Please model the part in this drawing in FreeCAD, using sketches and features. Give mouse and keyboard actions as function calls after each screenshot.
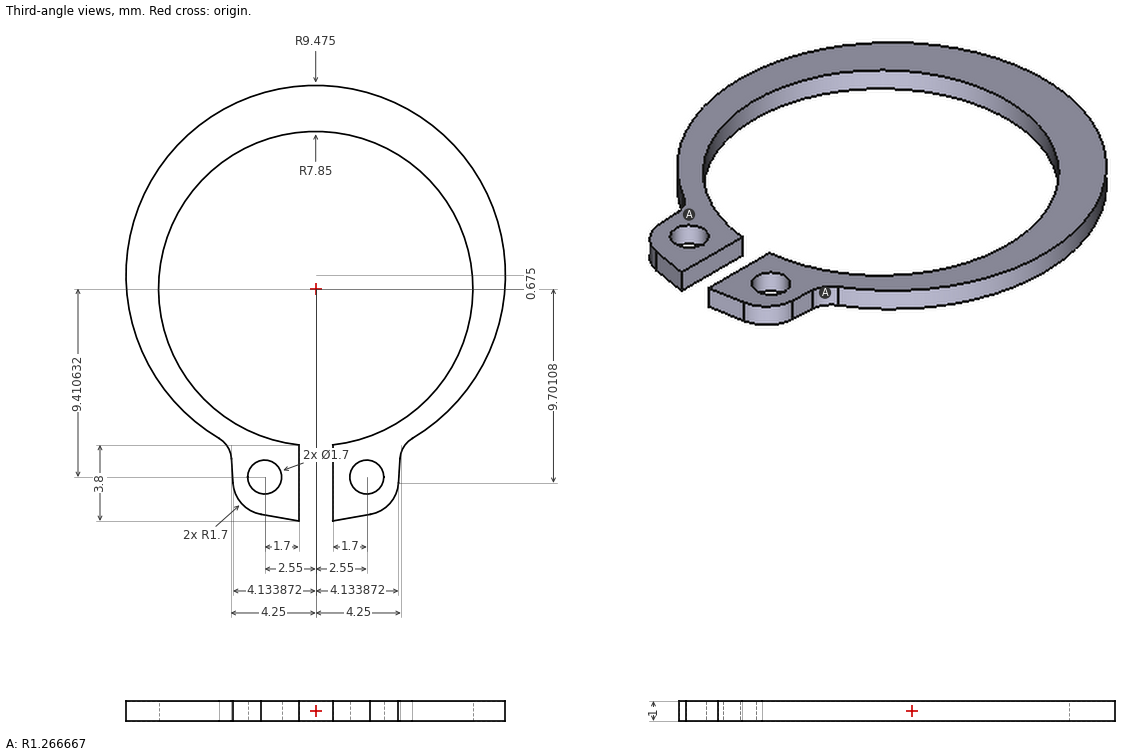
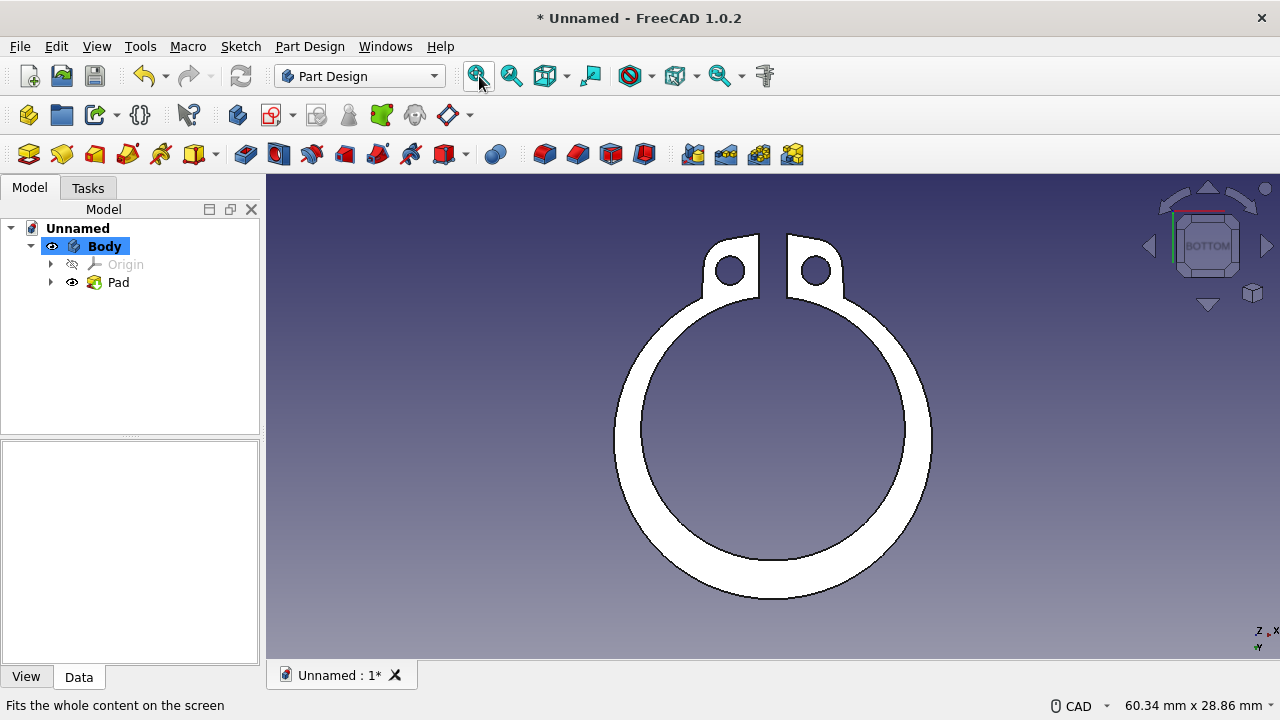
key(4)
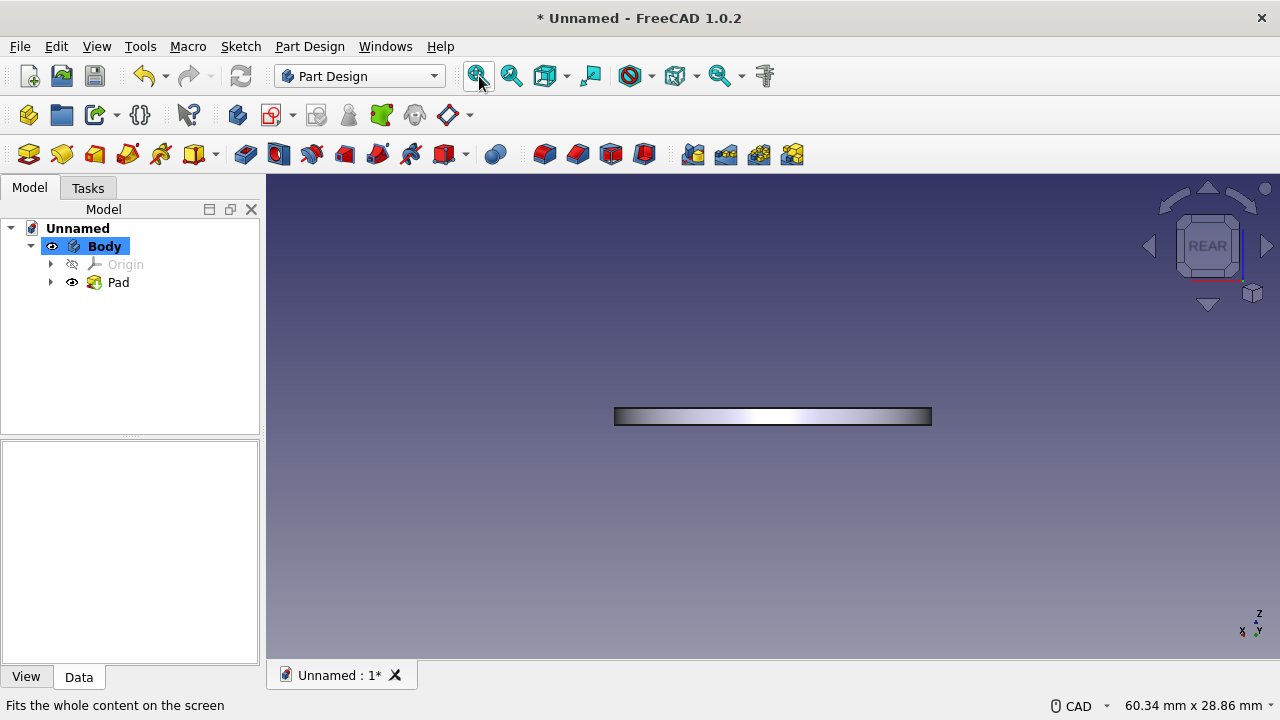
click(479, 76)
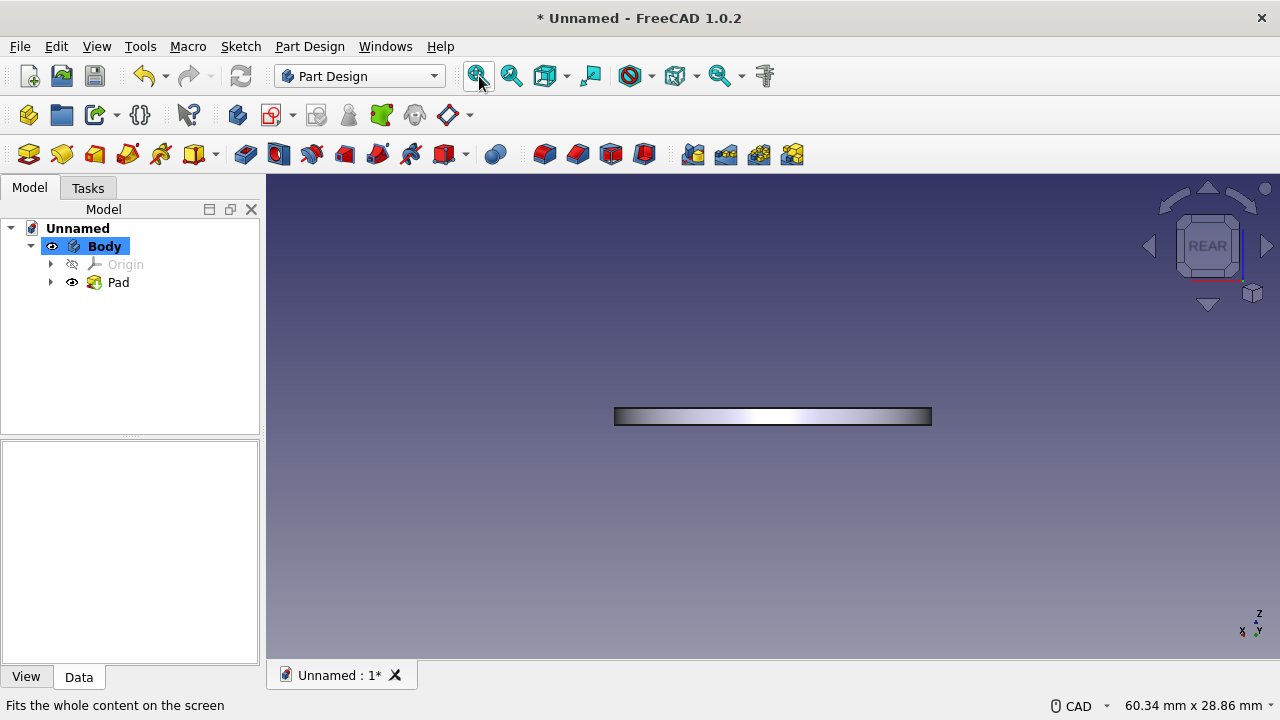
scroll(844, 416, up, 5)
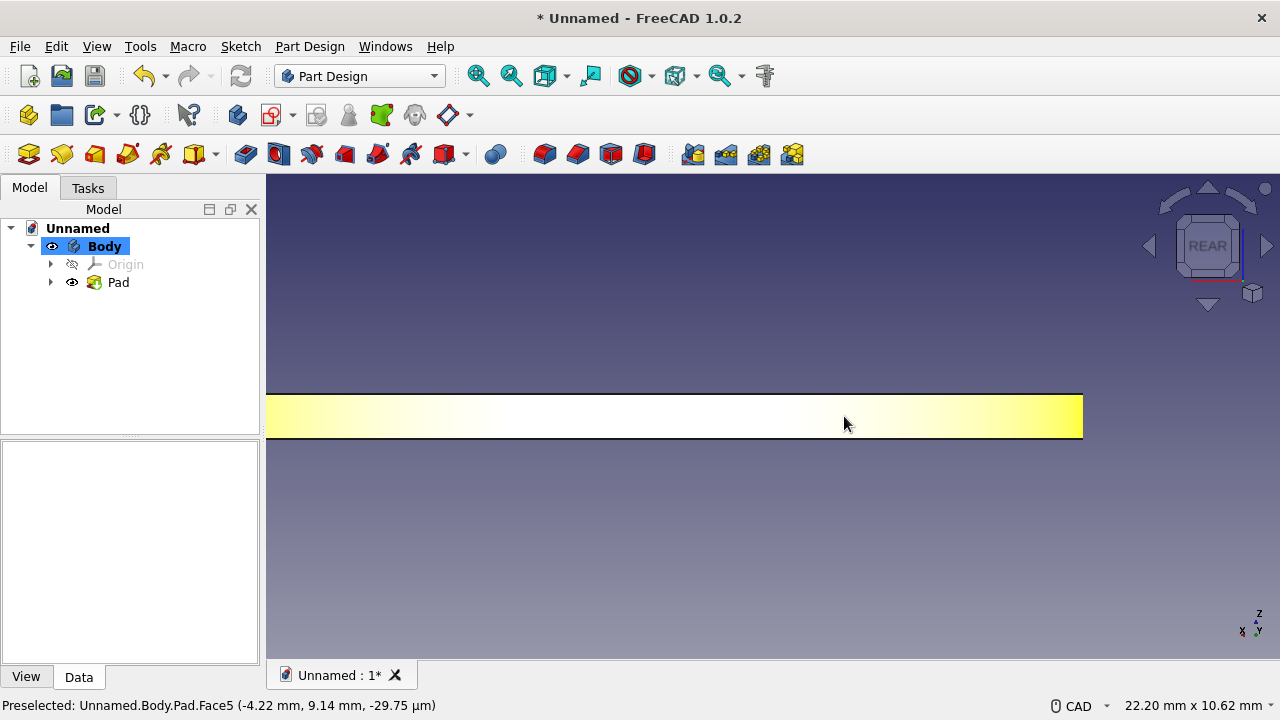
click(479, 76)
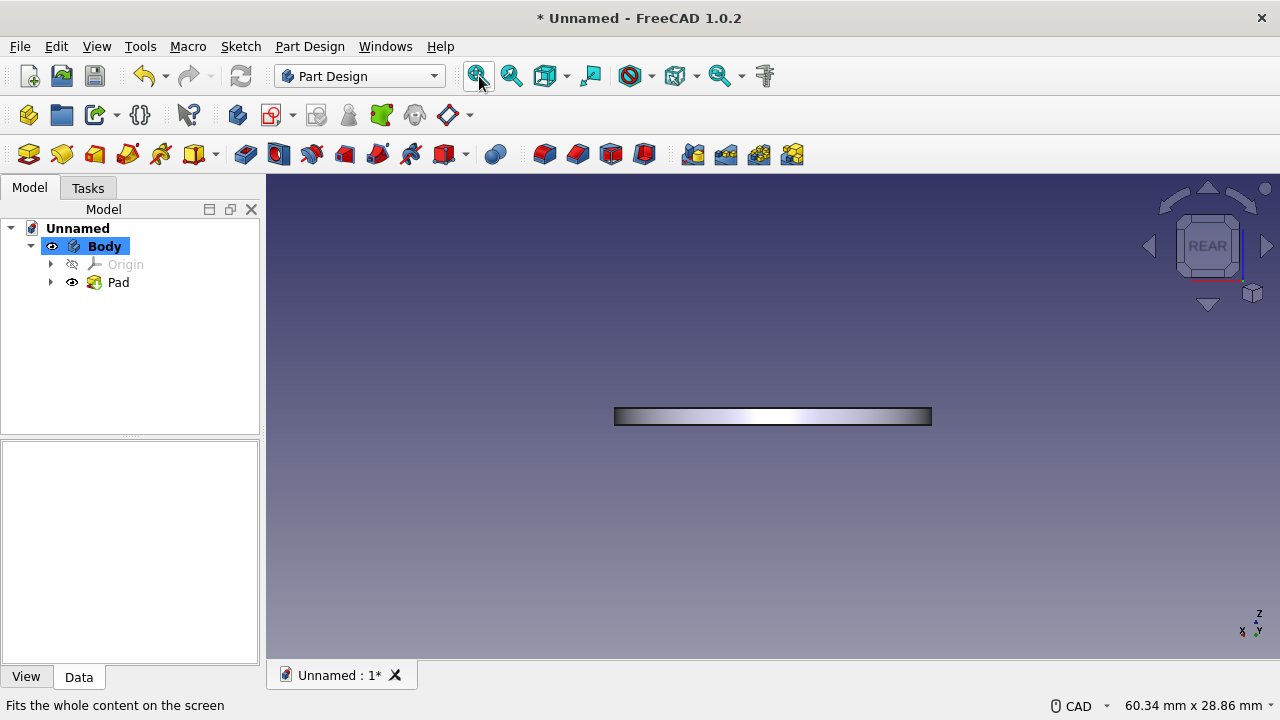
key(6)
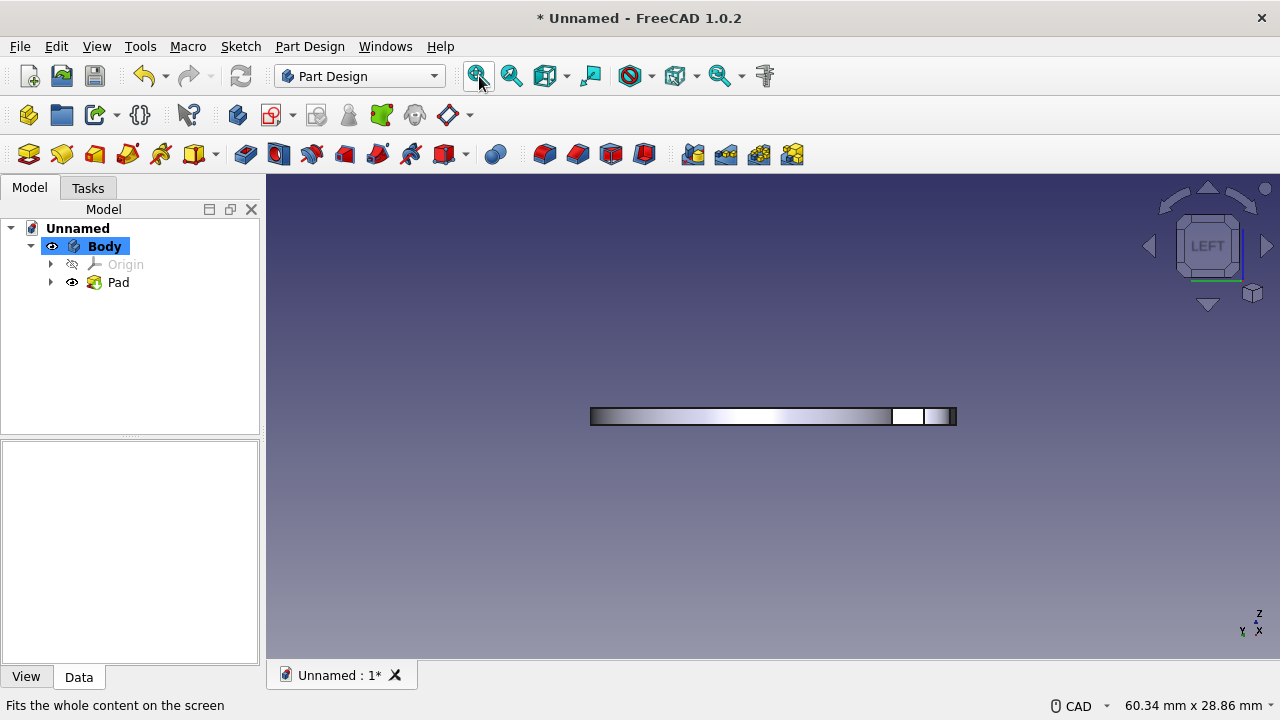
click(479, 76)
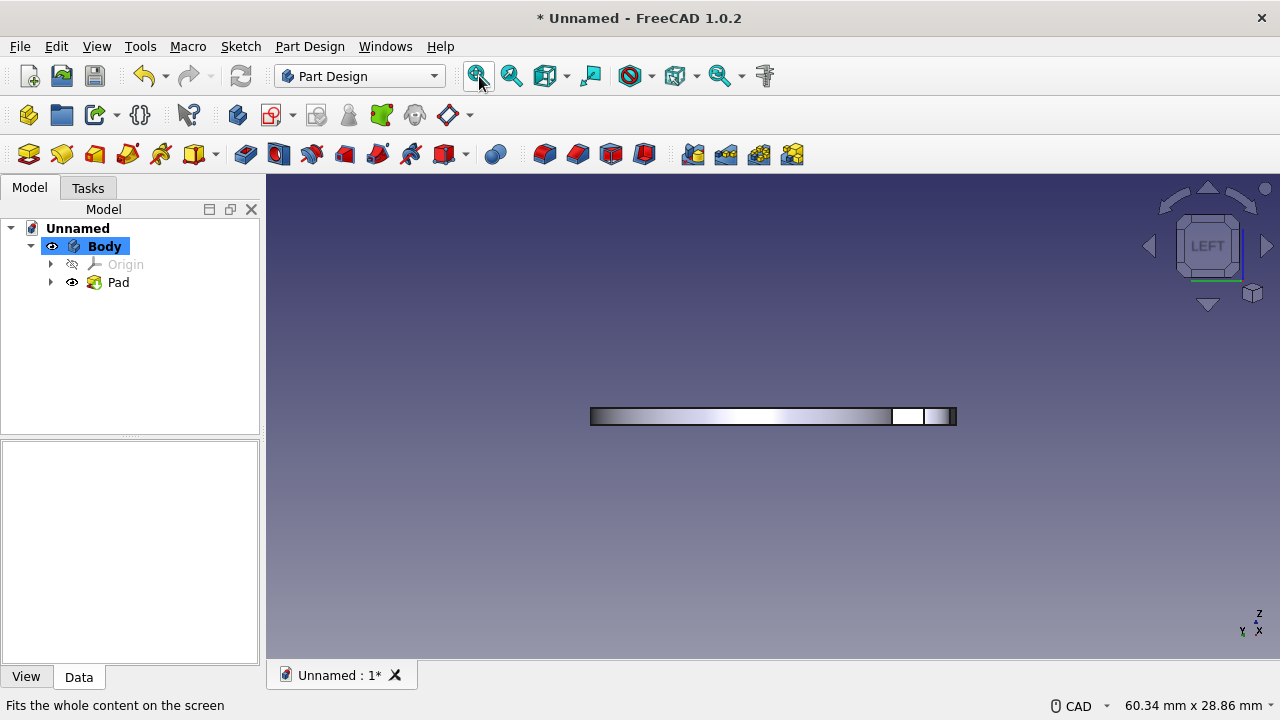
scroll(892, 415, up, 5)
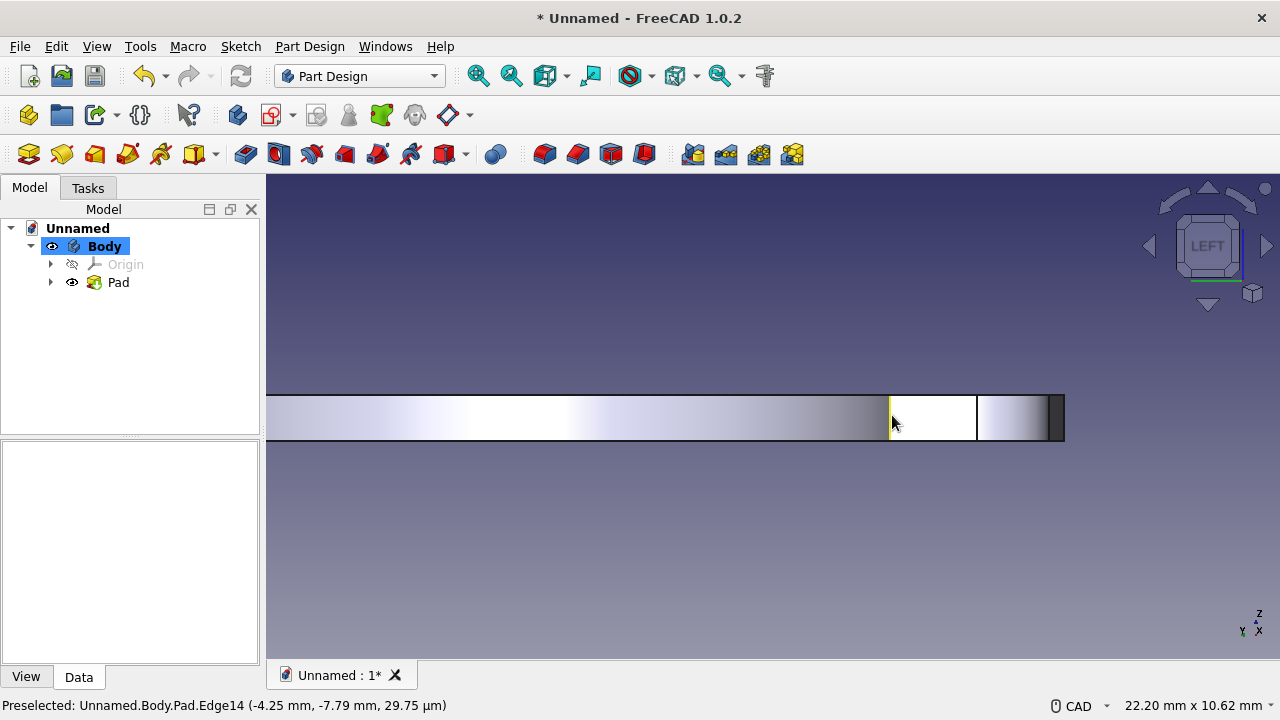
click(479, 76)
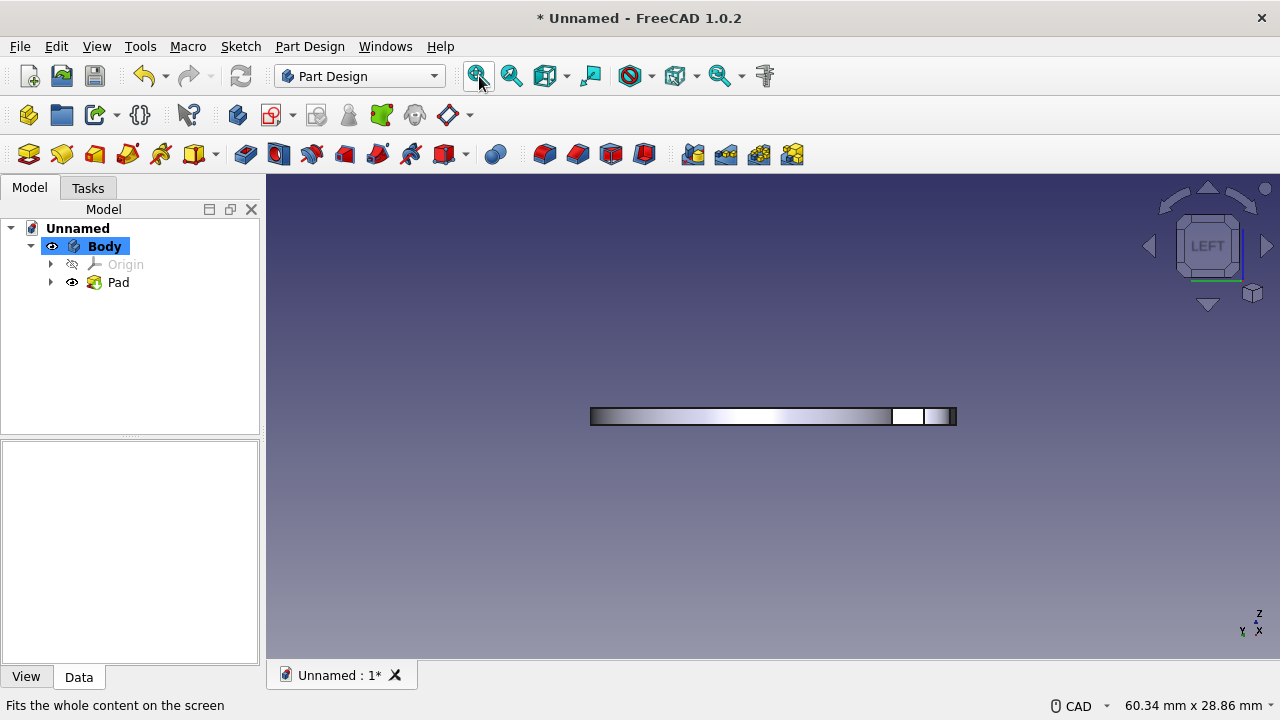
key(v)
key(3)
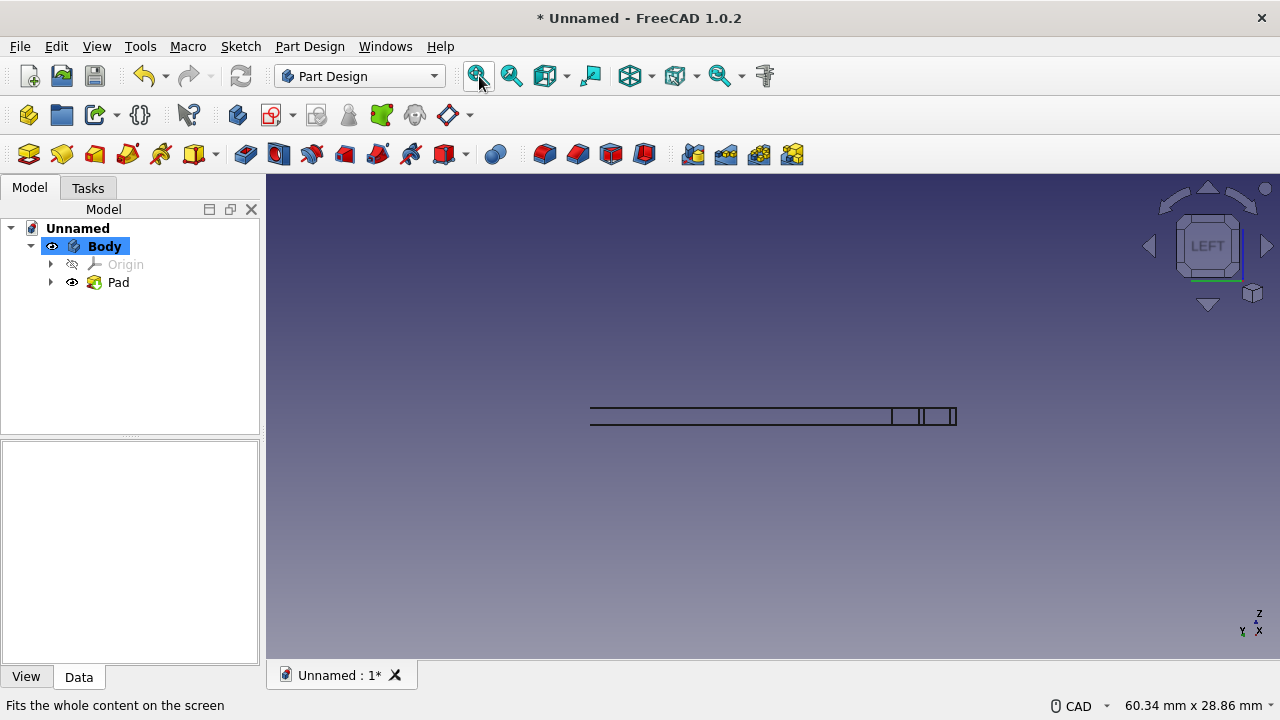
key(0)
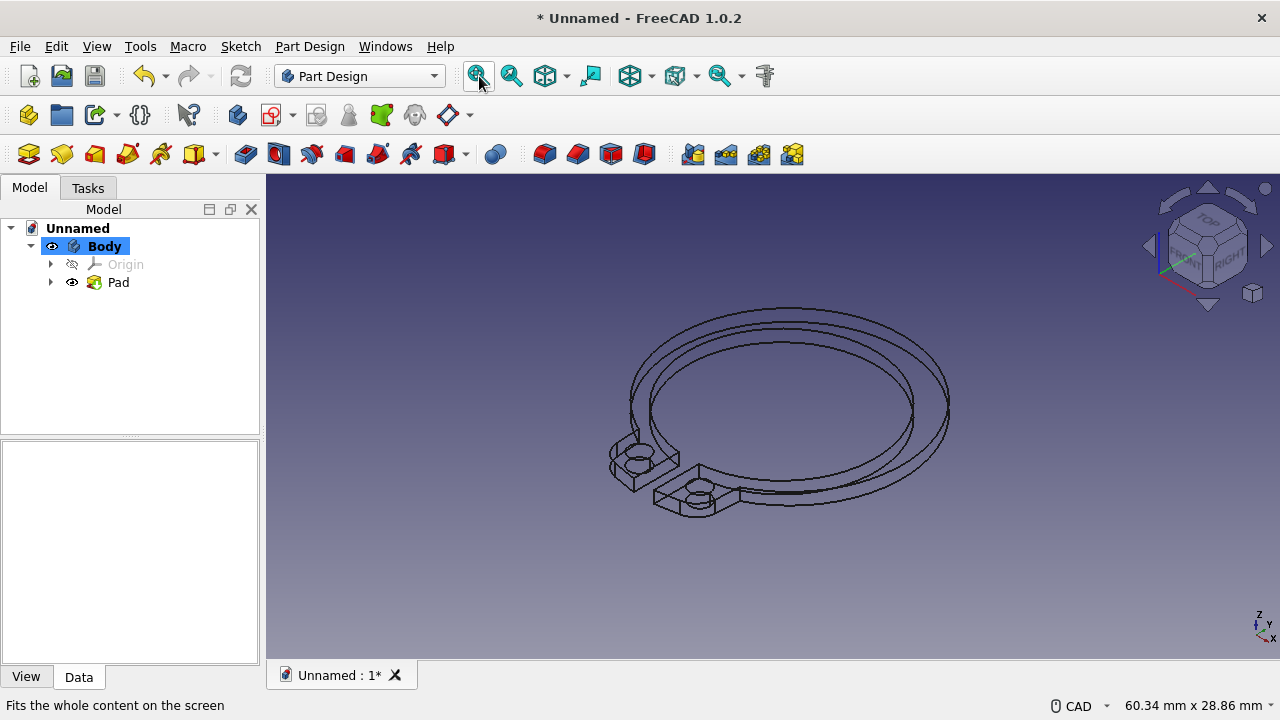
click(639, 436)